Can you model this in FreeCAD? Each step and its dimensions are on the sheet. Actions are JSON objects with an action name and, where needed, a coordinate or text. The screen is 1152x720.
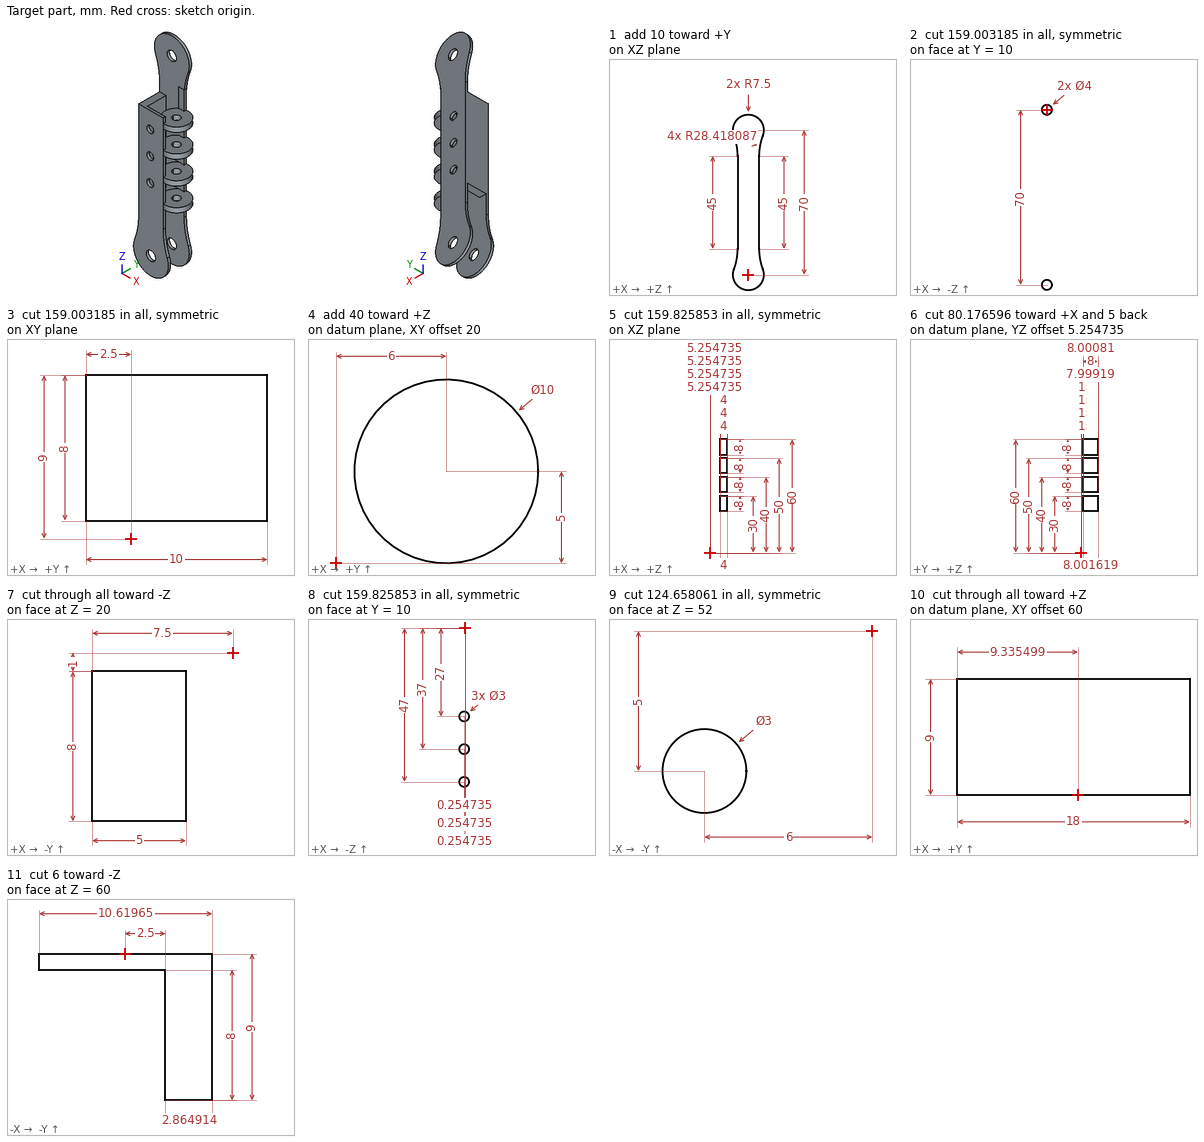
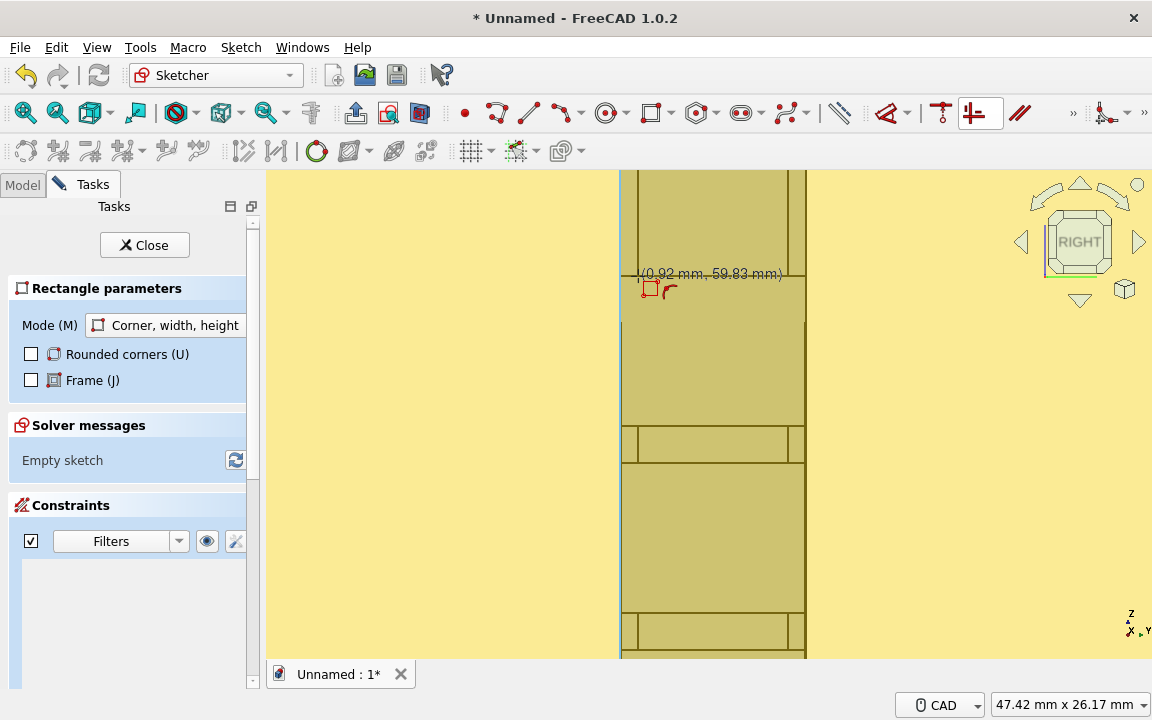
{"action": "left_click", "coordinate": [638, 276]}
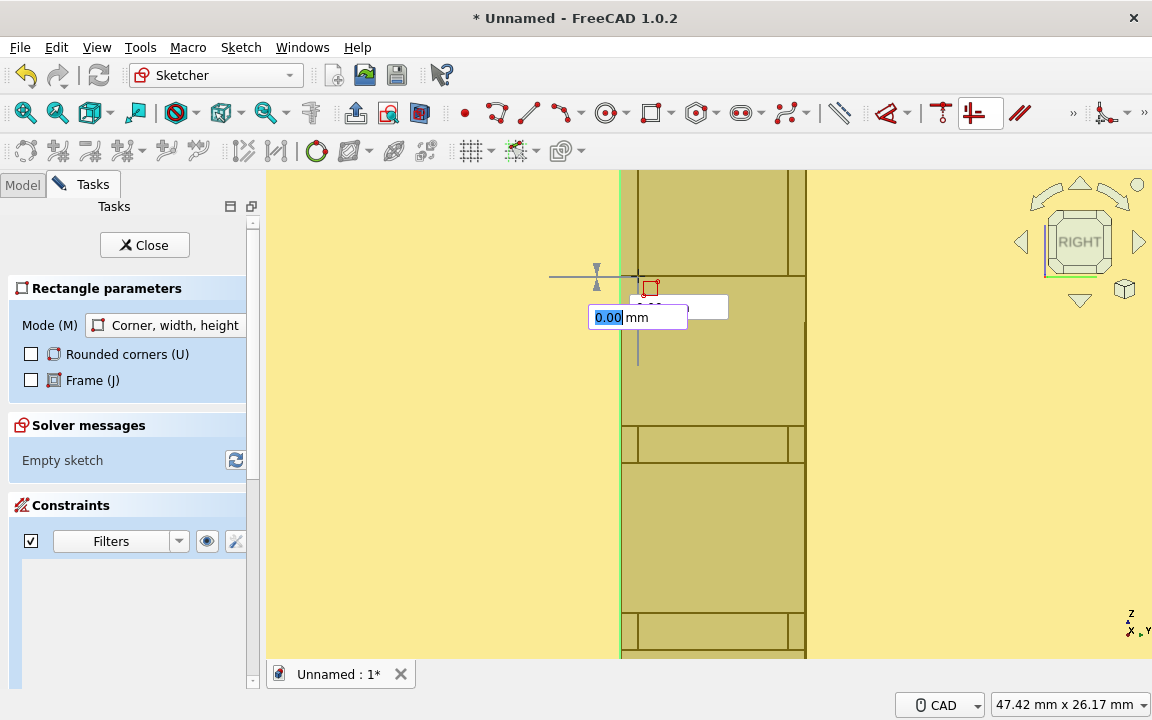
{"action": "scroll", "coordinate": [613, 232], "scroll_direction": "down", "scroll_amount": 6}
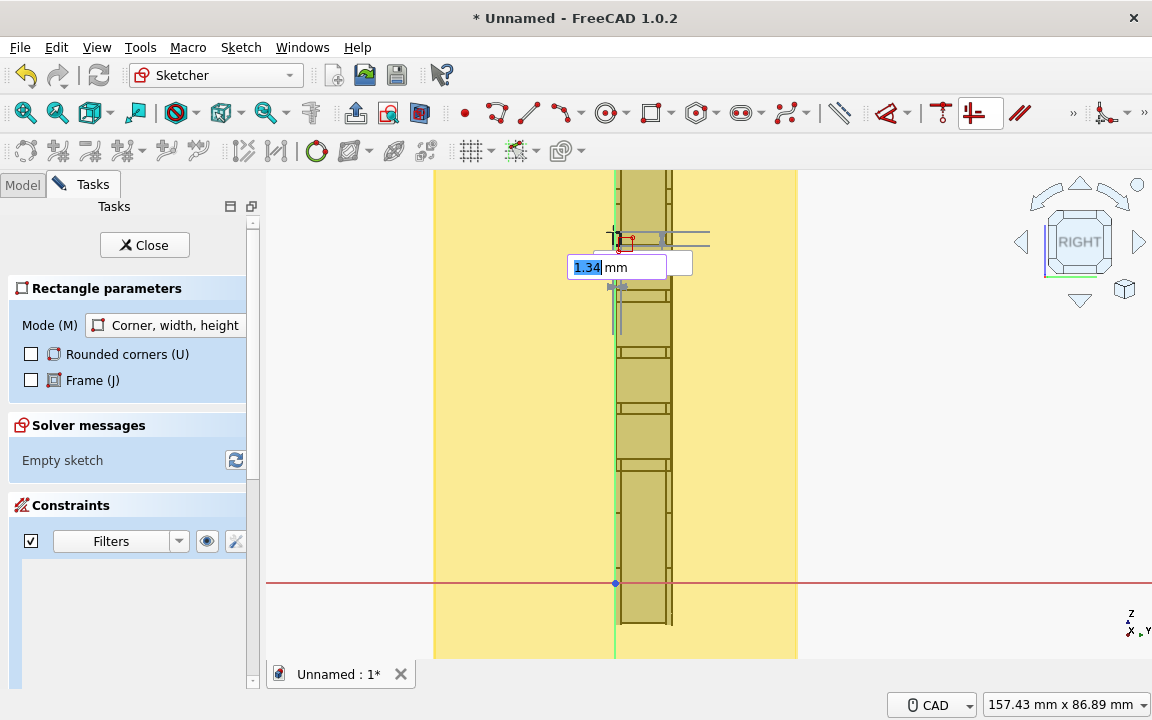
{"action": "left_click", "coordinate": [666, 290]}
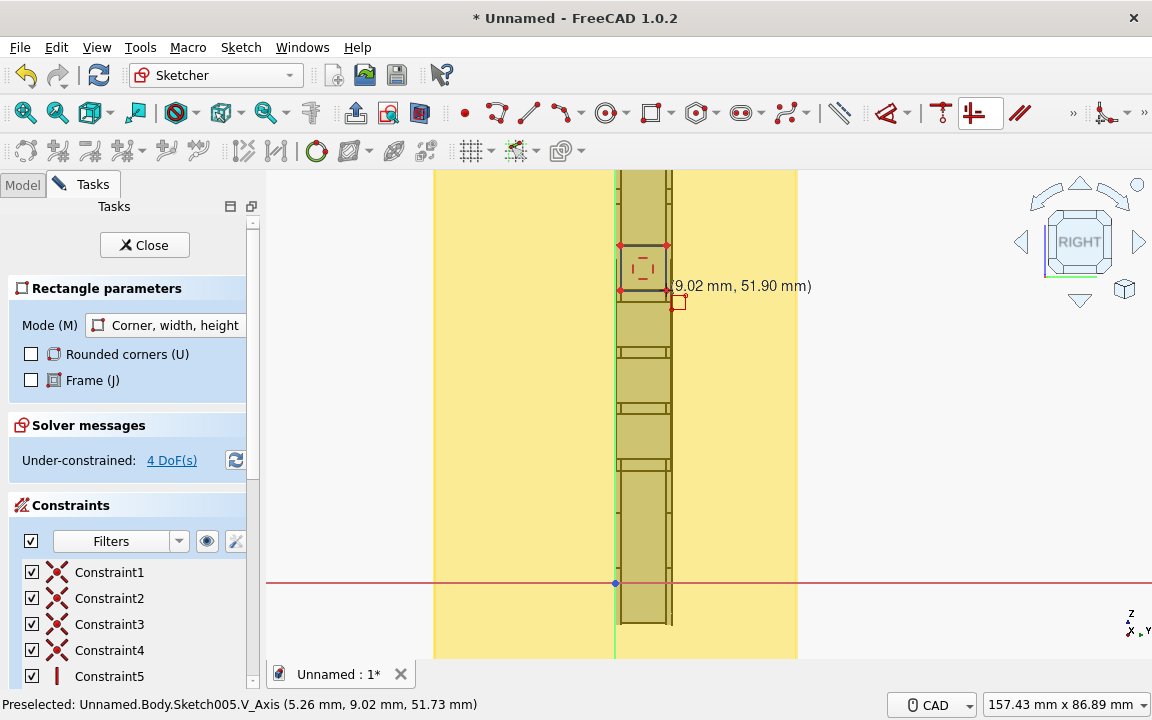
{"action": "scroll", "coordinate": [621, 302], "scroll_direction": "up", "scroll_amount": 6}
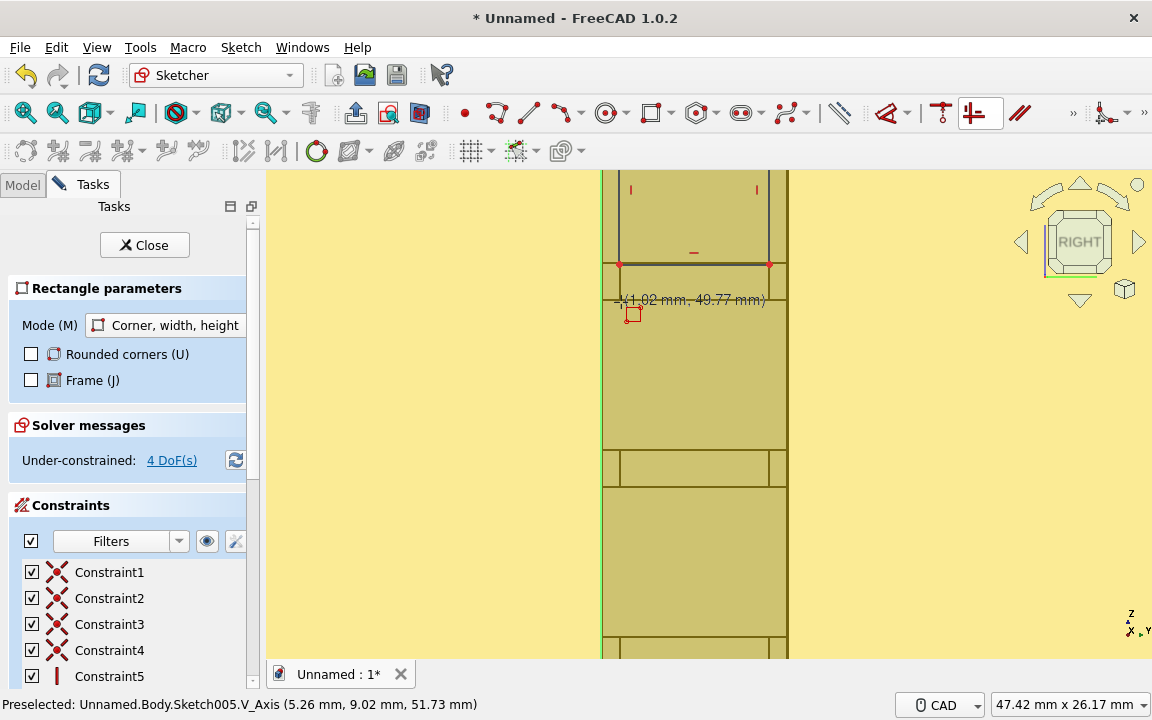
{"action": "left_click", "coordinate": [620, 300]}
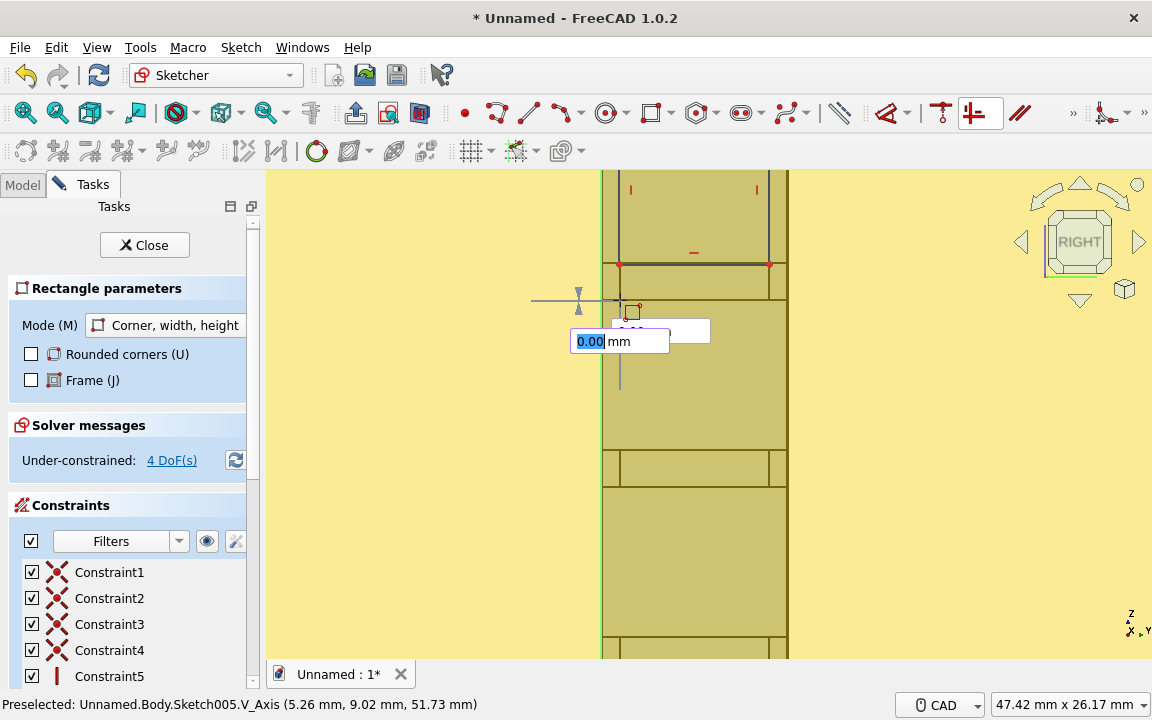
{"action": "scroll", "coordinate": [621, 303], "scroll_direction": "down", "scroll_amount": 6}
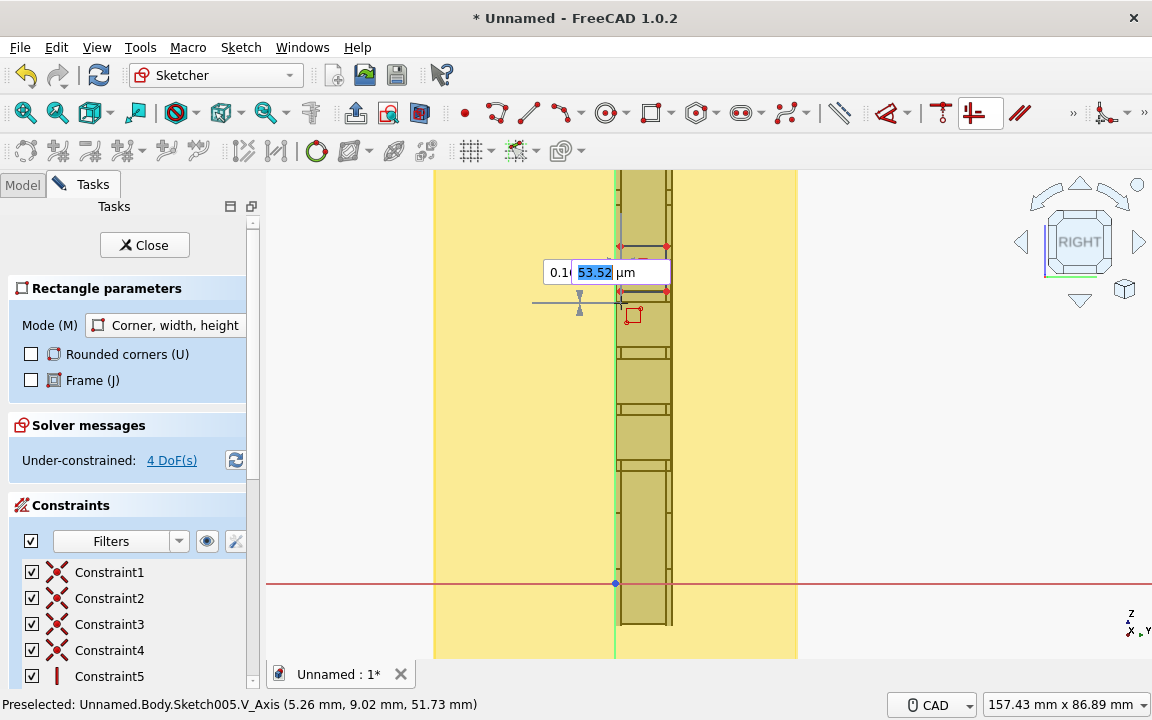
{"action": "left_click", "coordinate": [666, 347]}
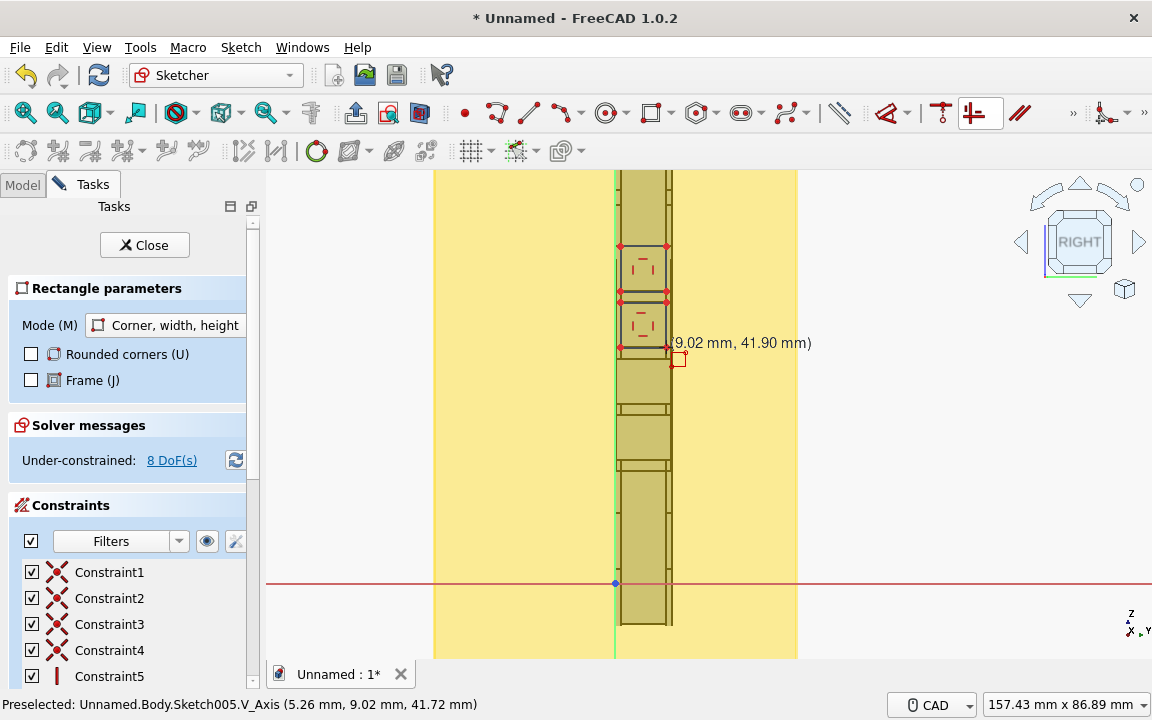
{"action": "scroll", "coordinate": [621, 359], "scroll_direction": "up", "scroll_amount": 6}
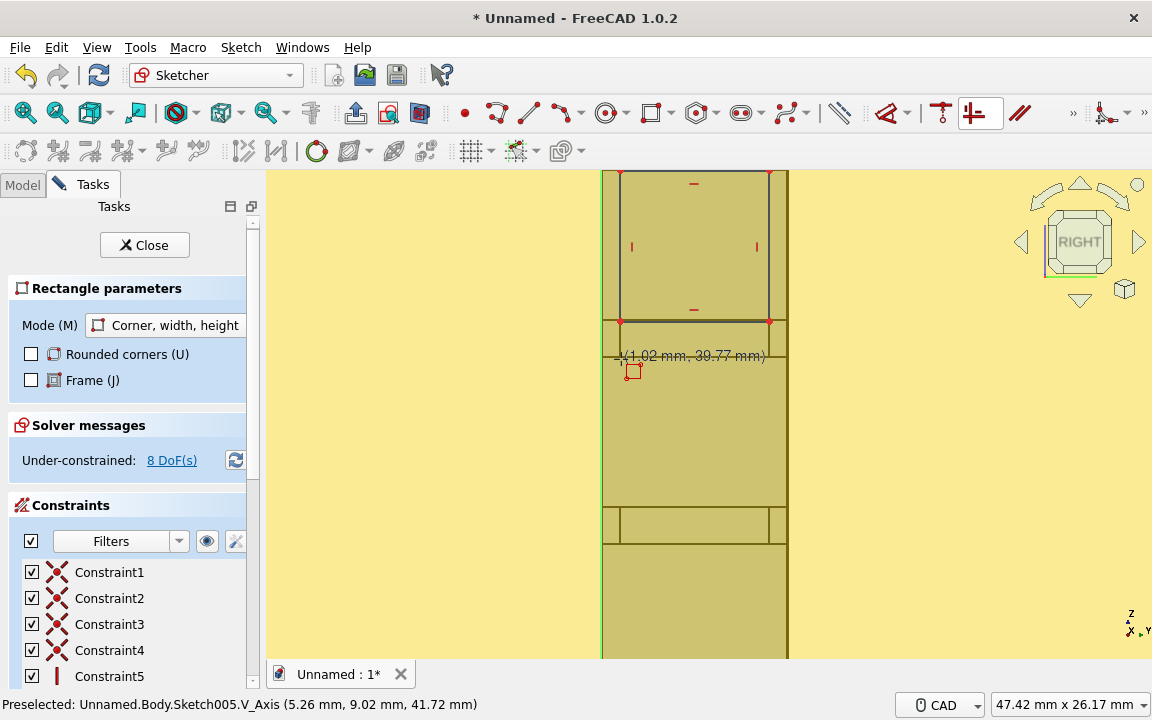
{"action": "left_click", "coordinate": [620, 357]}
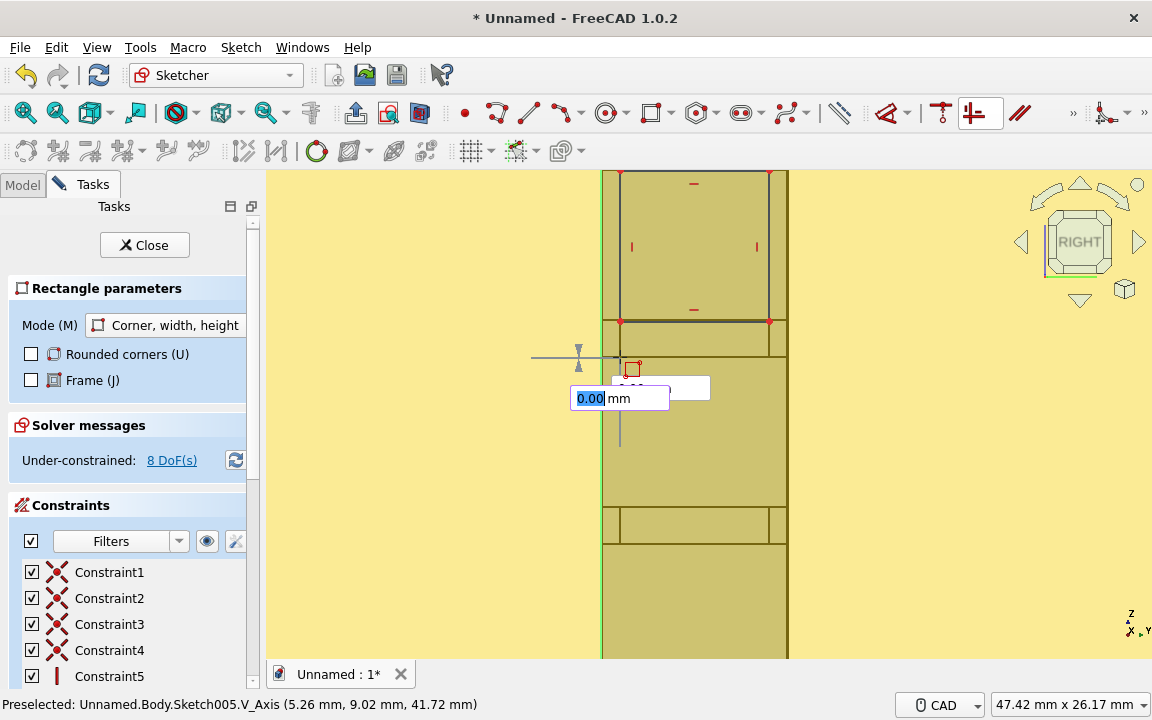
{"action": "scroll", "coordinate": [621, 359], "scroll_direction": "down", "scroll_amount": 6}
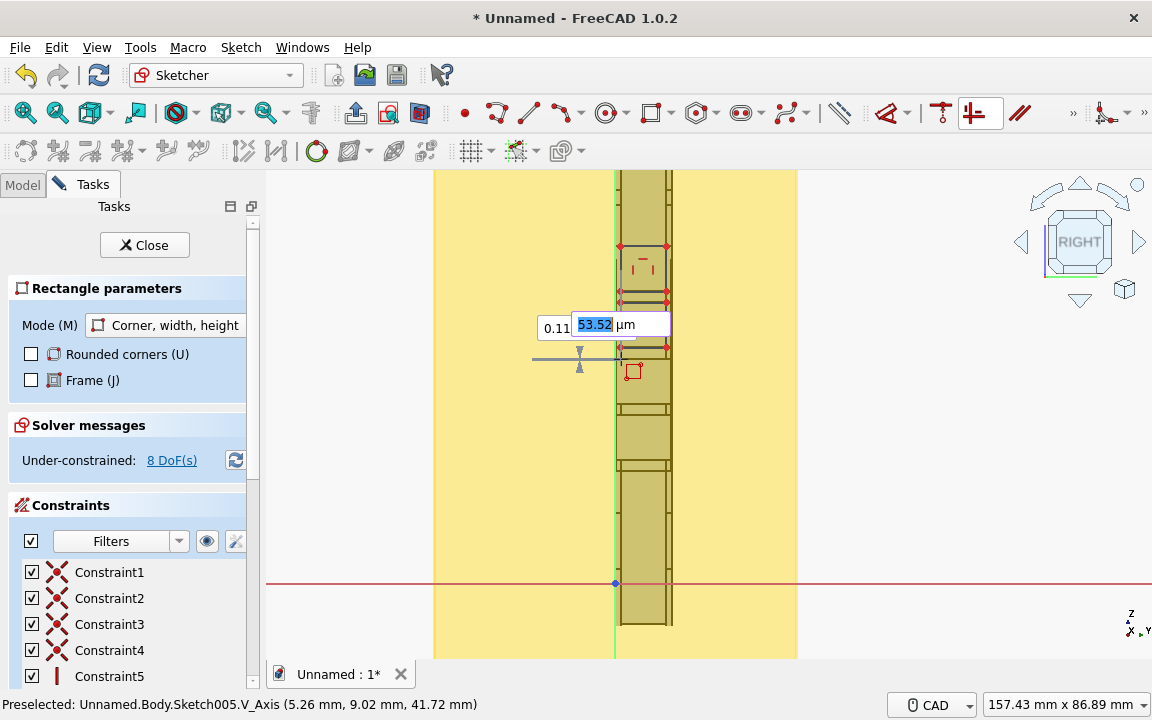
{"action": "left_click", "coordinate": [666, 404]}